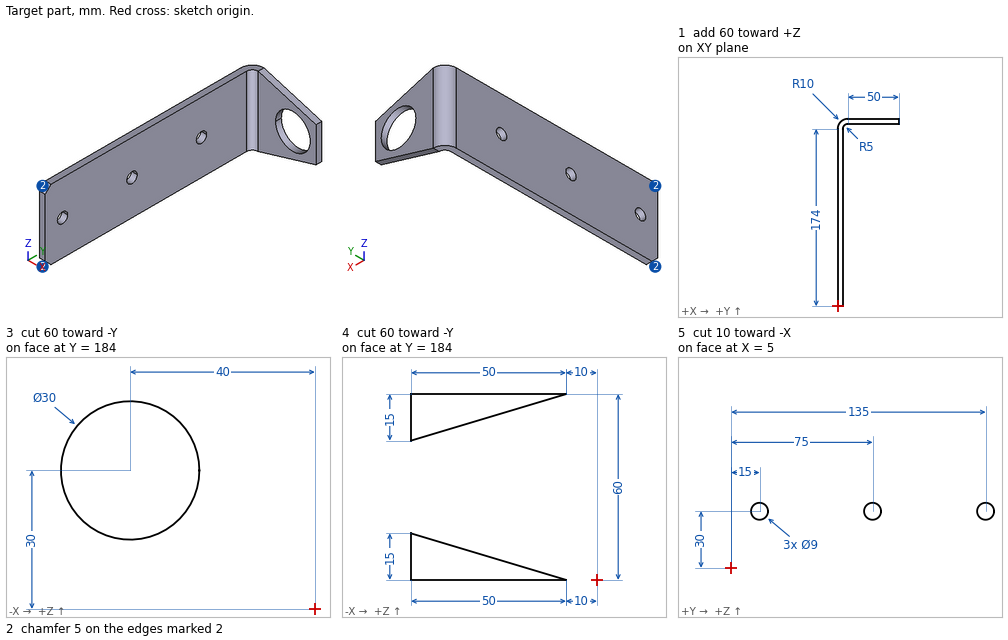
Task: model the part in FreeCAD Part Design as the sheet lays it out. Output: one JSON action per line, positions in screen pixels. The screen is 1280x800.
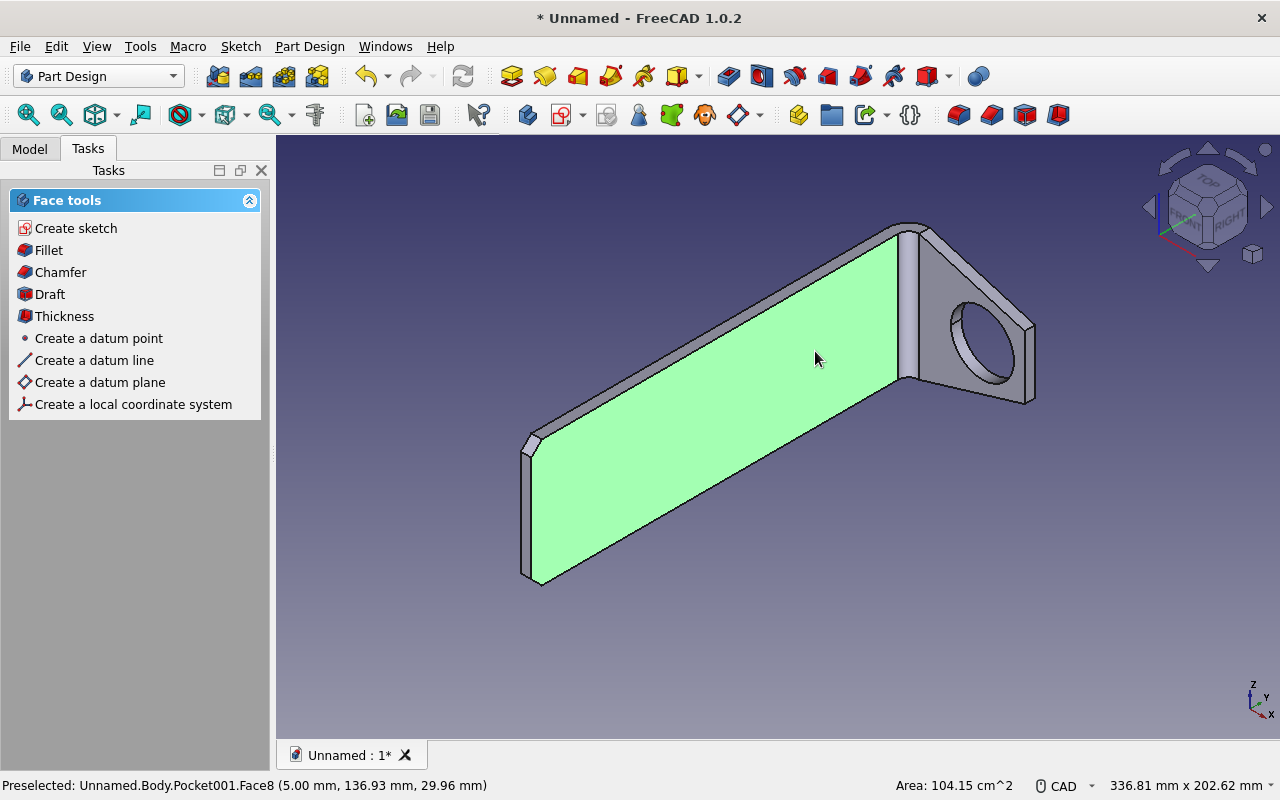
{"action": "left_click", "coordinate": [560, 116]}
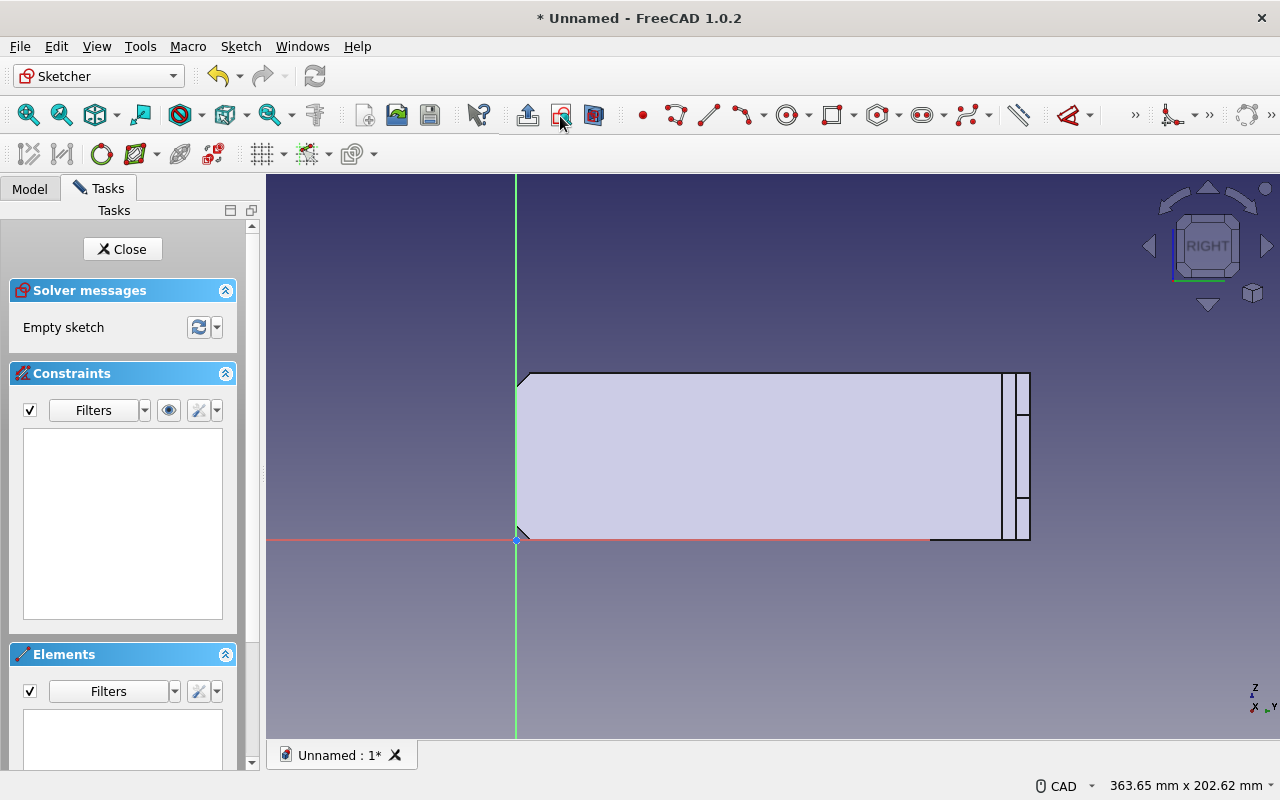
{"action": "scroll", "coordinate": [724, 564], "scroll_direction": "up", "scroll_amount": 2}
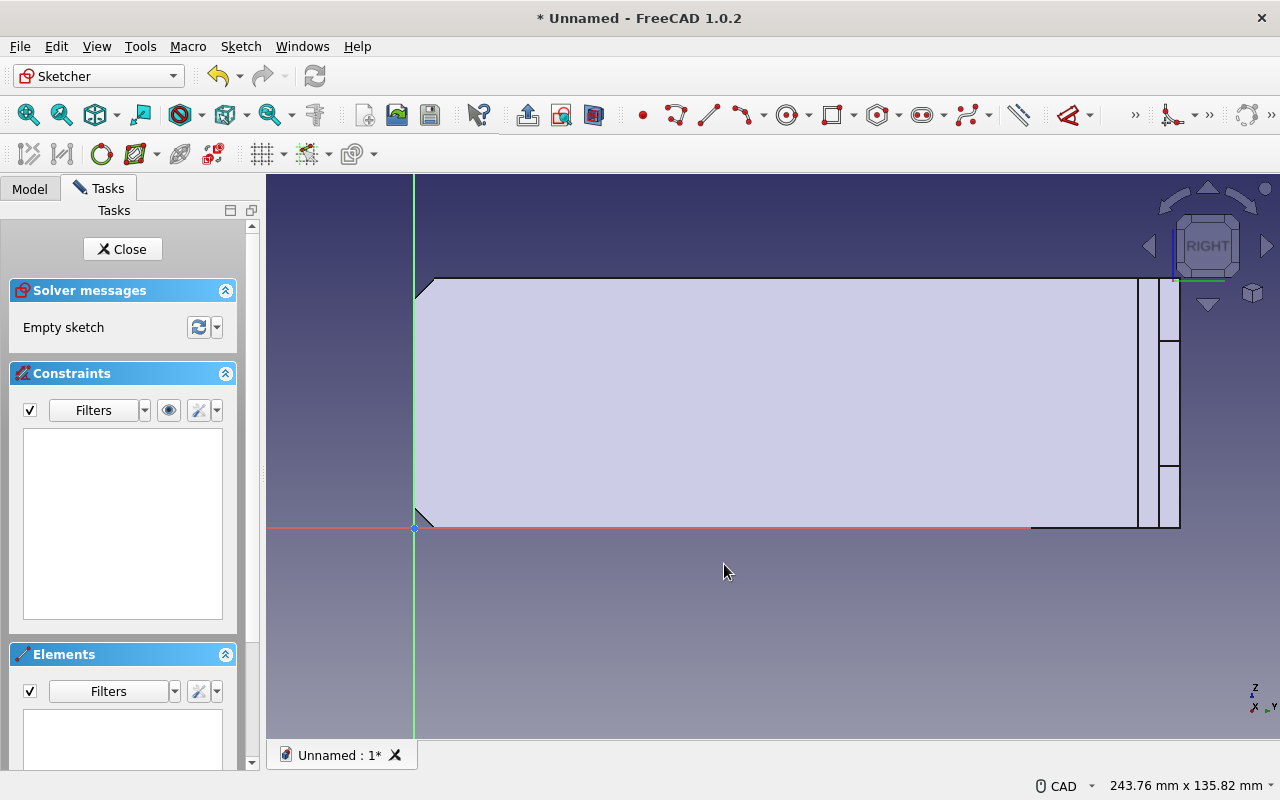
{"action": "key", "text": "g c"}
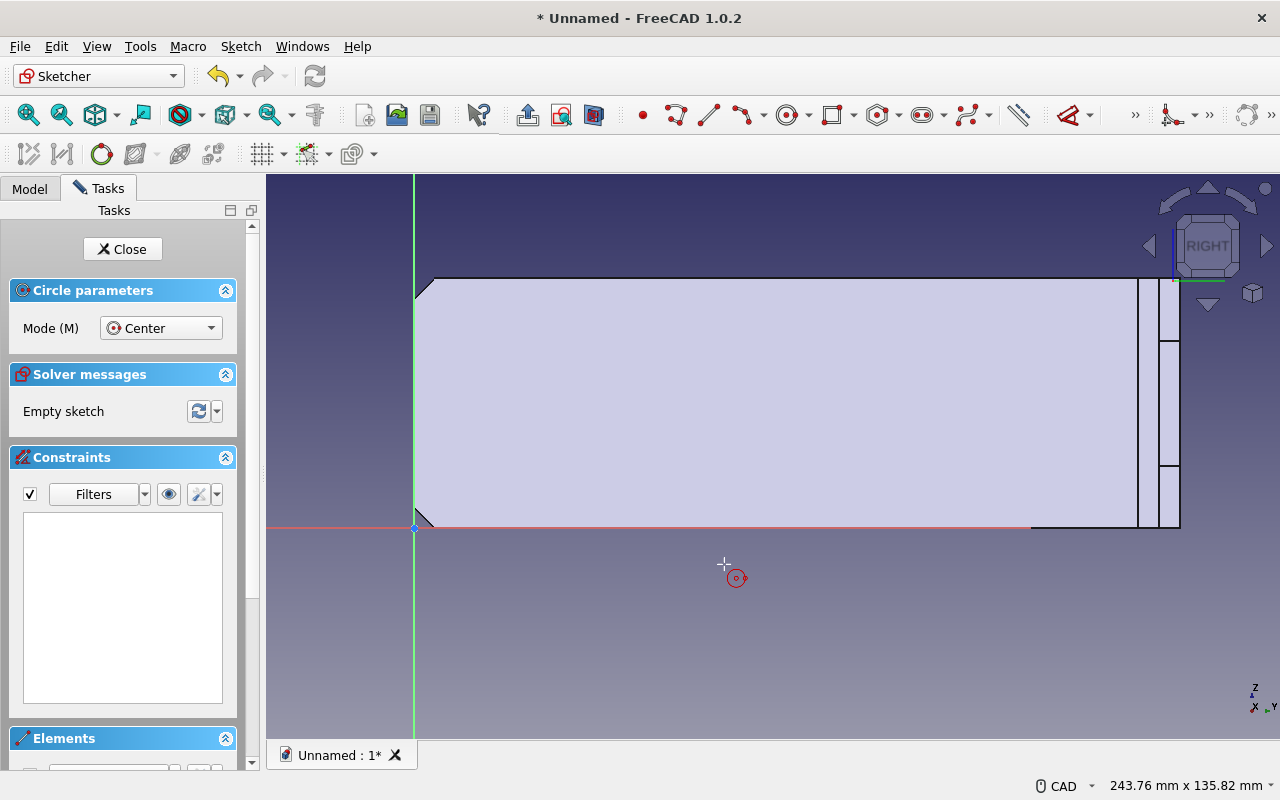
{"action": "left_click", "coordinate": [477, 403]}
{"action": "left_click", "coordinate": [490, 390]}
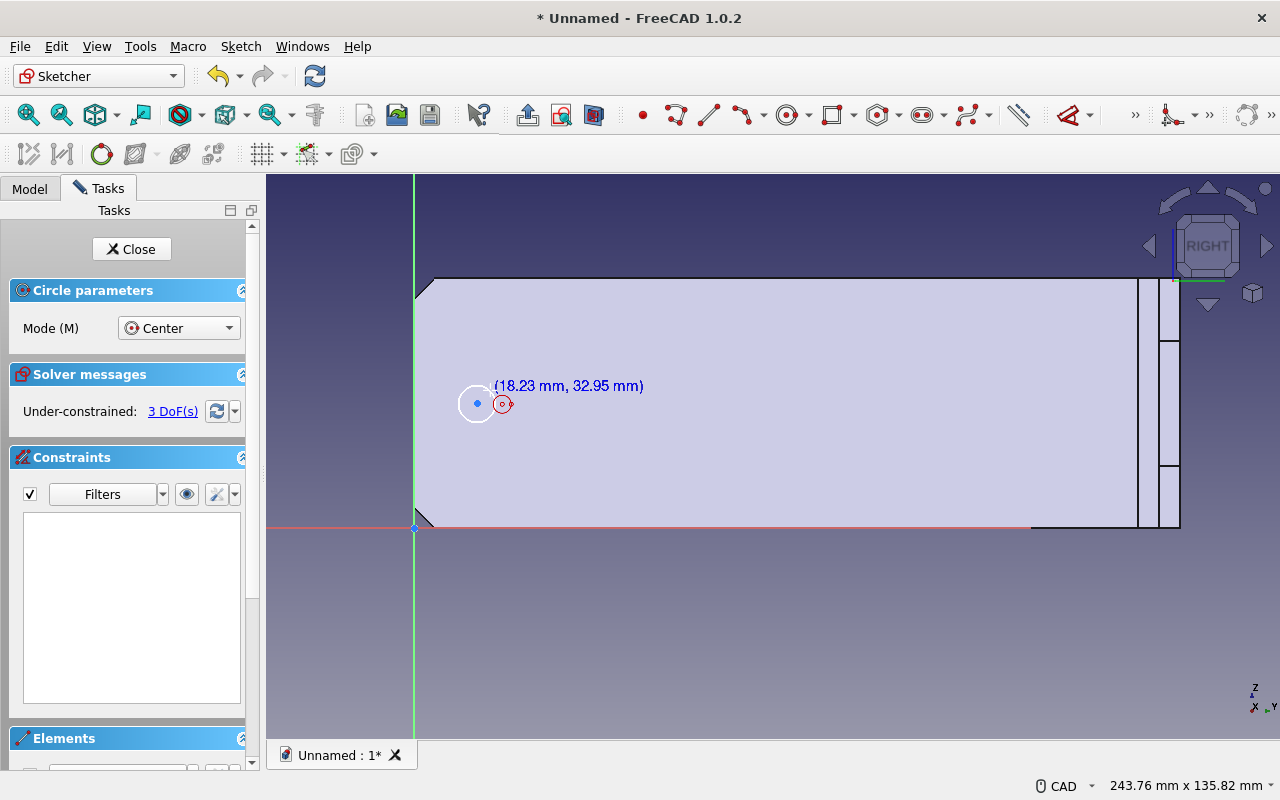
{"action": "left_click", "coordinate": [726, 403]}
{"action": "left_click", "coordinate": [739, 390]}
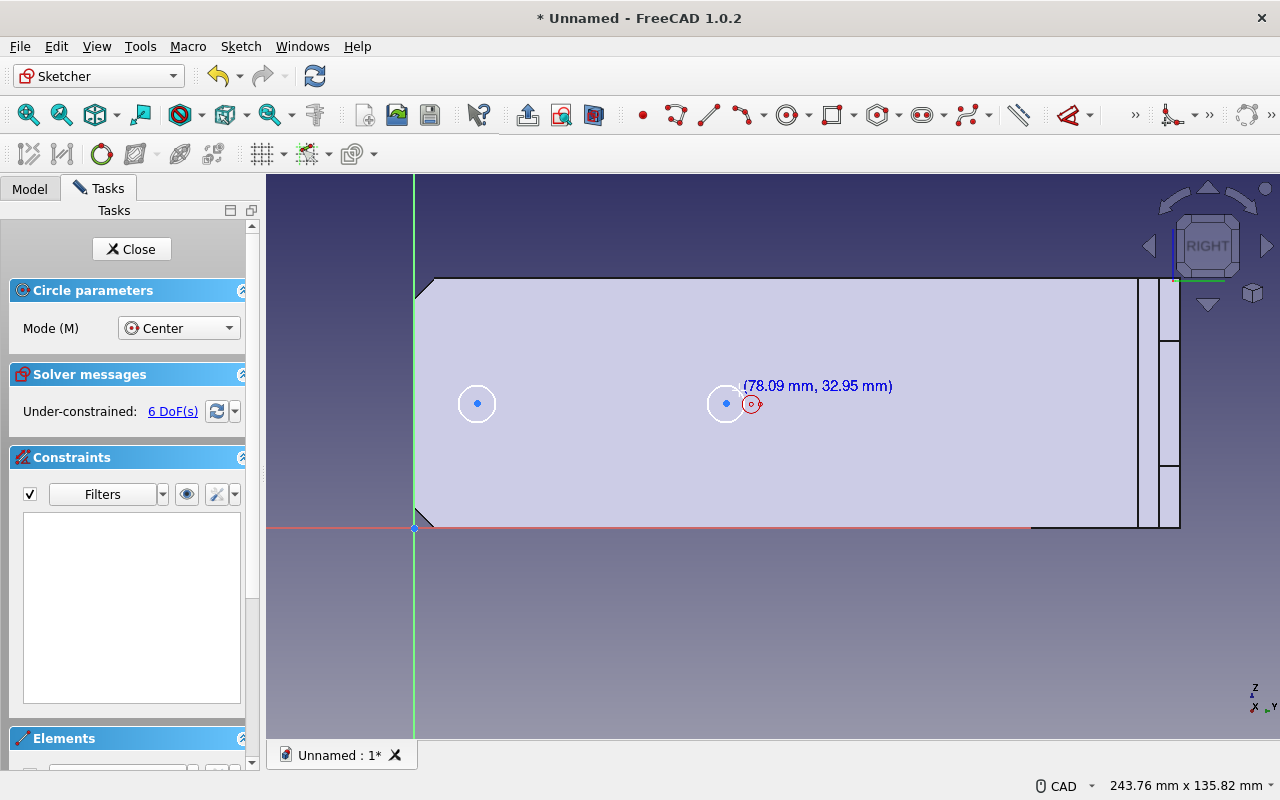
{"action": "left_click", "coordinate": [976, 403]}
{"action": "left_click", "coordinate": [989, 390]}
{"action": "key", "text": "Escape"}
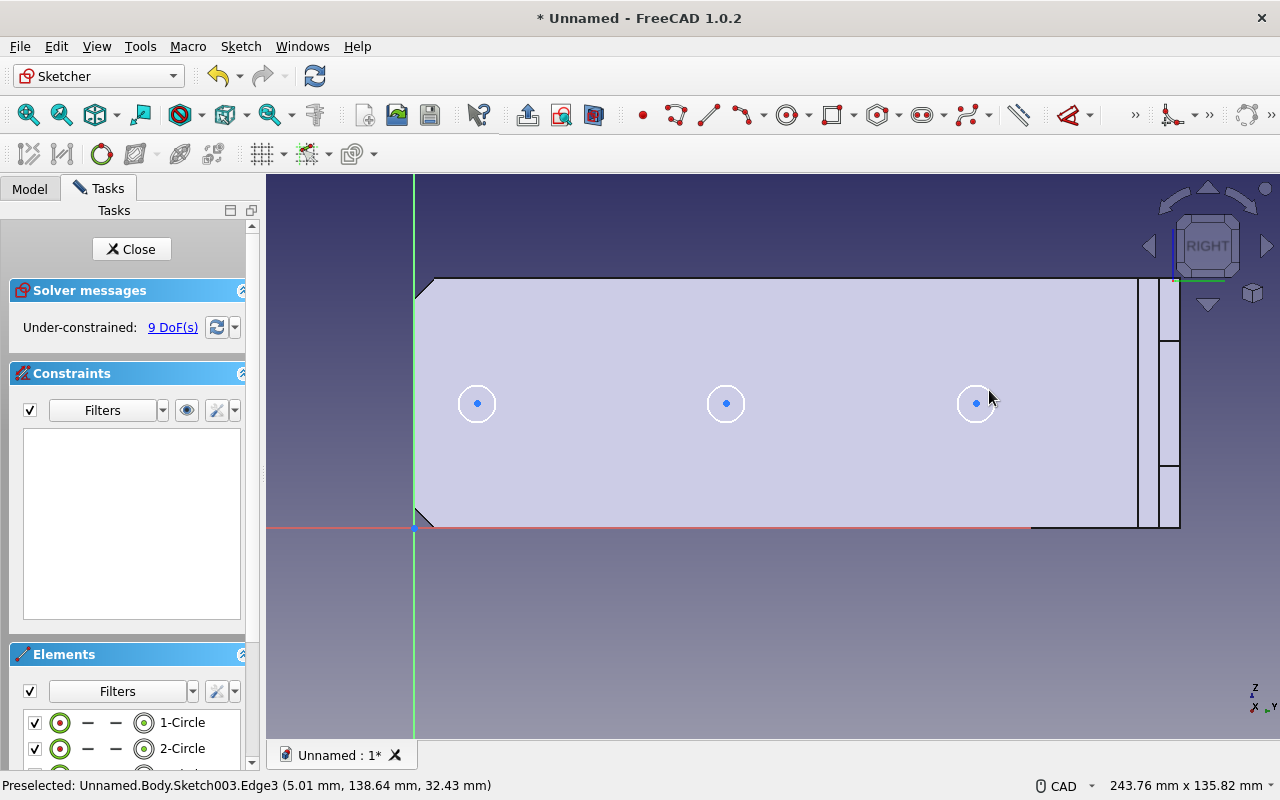
{"action": "left_click", "coordinate": [490, 391]}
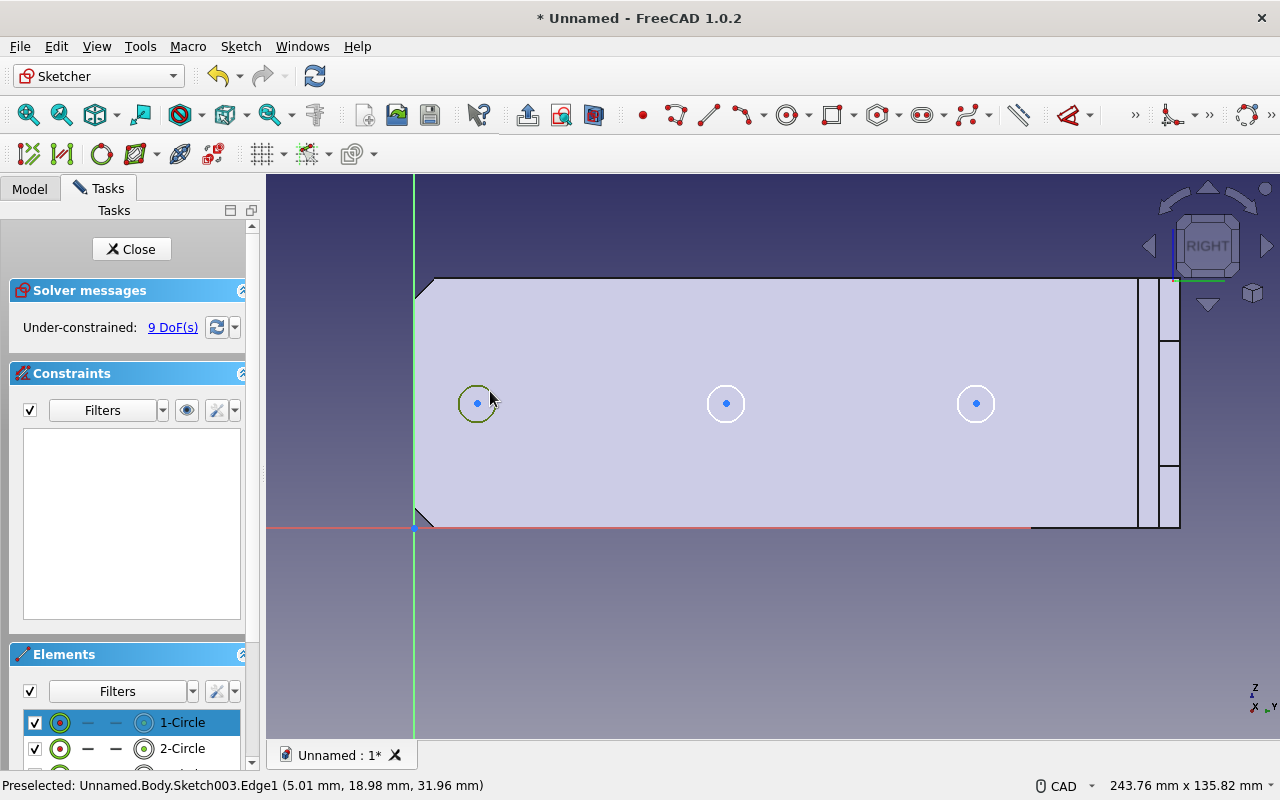
{"action": "left_click", "coordinate": [739, 391]}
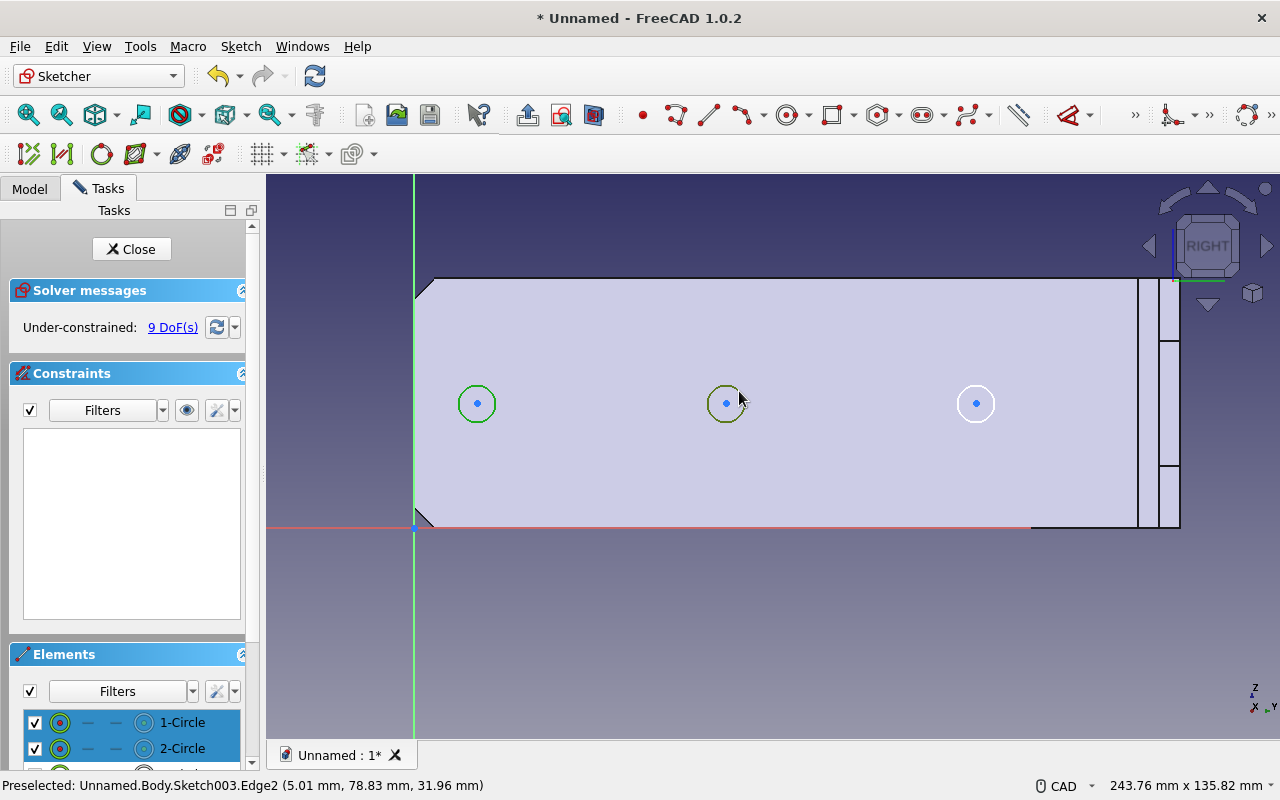
{"action": "left_click", "coordinate": [989, 391]}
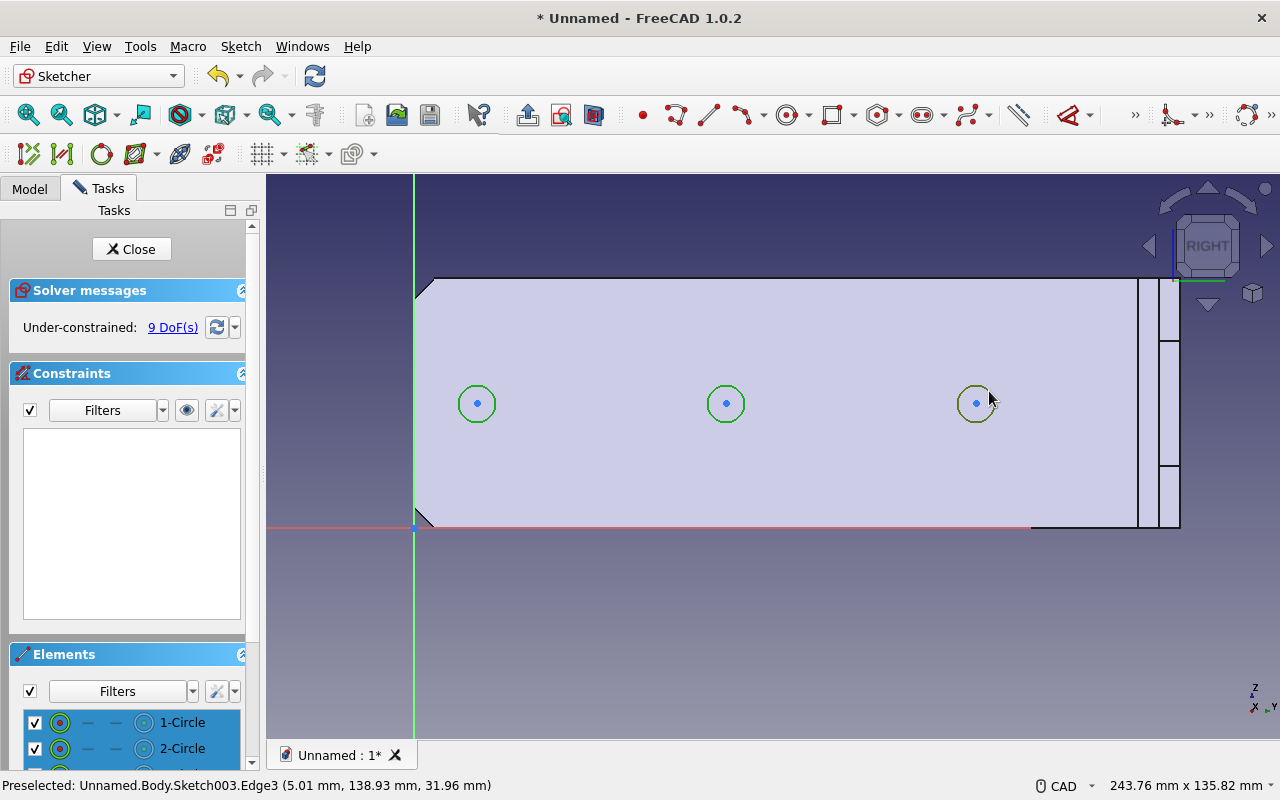
{"action": "key", "text": "e"}